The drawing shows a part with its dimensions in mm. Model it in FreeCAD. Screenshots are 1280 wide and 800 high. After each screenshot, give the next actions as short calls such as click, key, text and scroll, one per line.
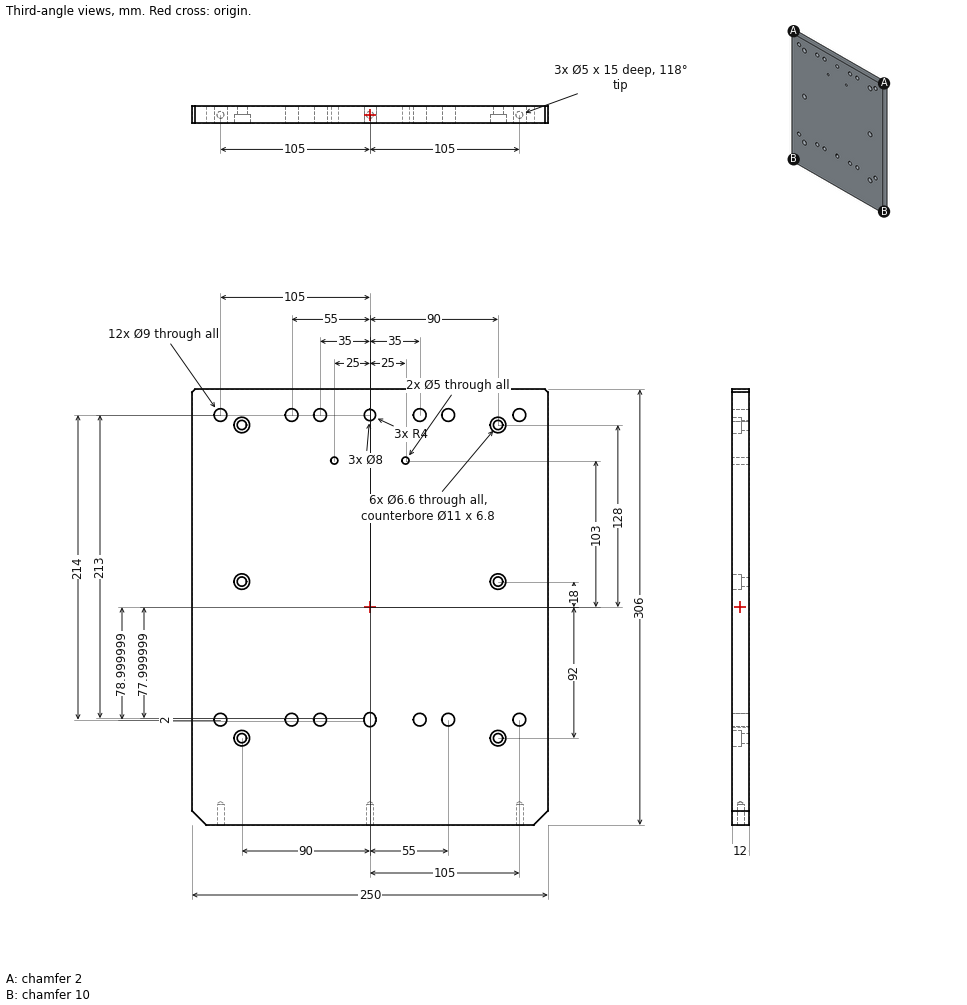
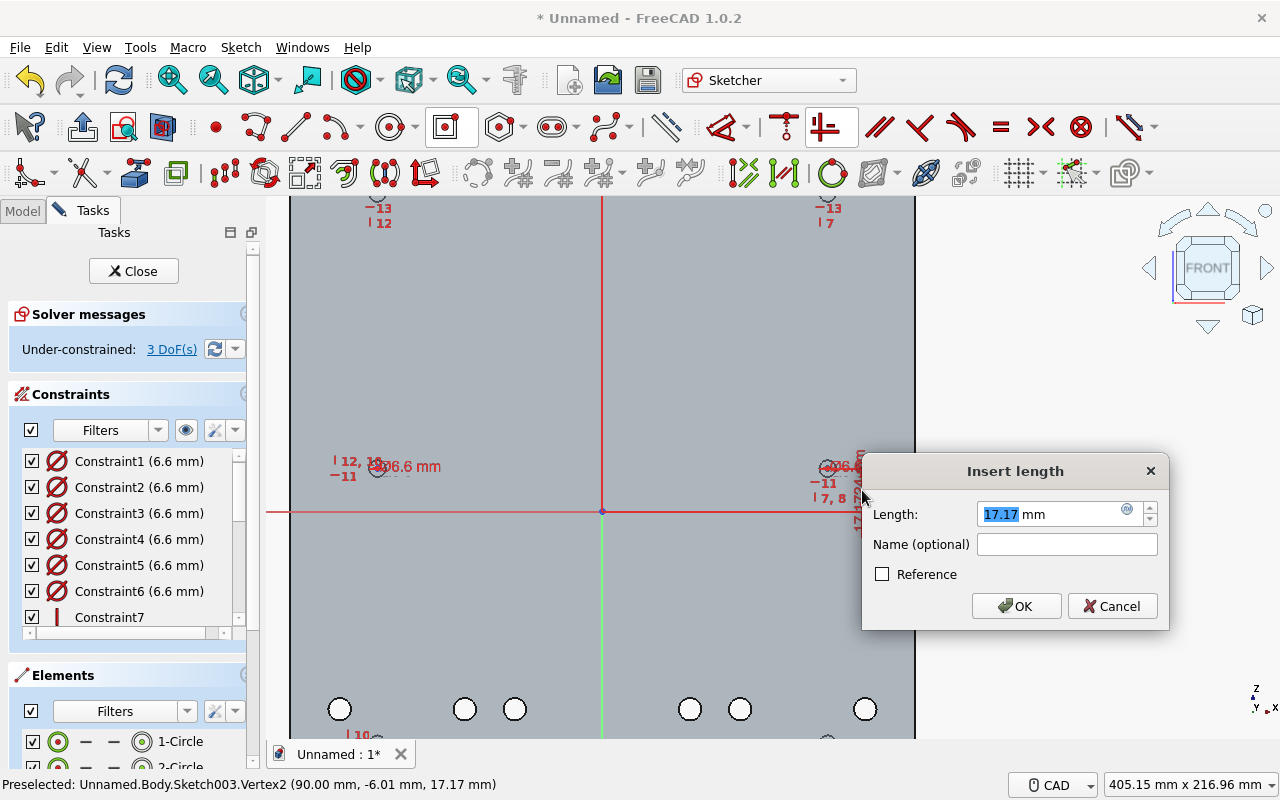
text(18)
key(Return)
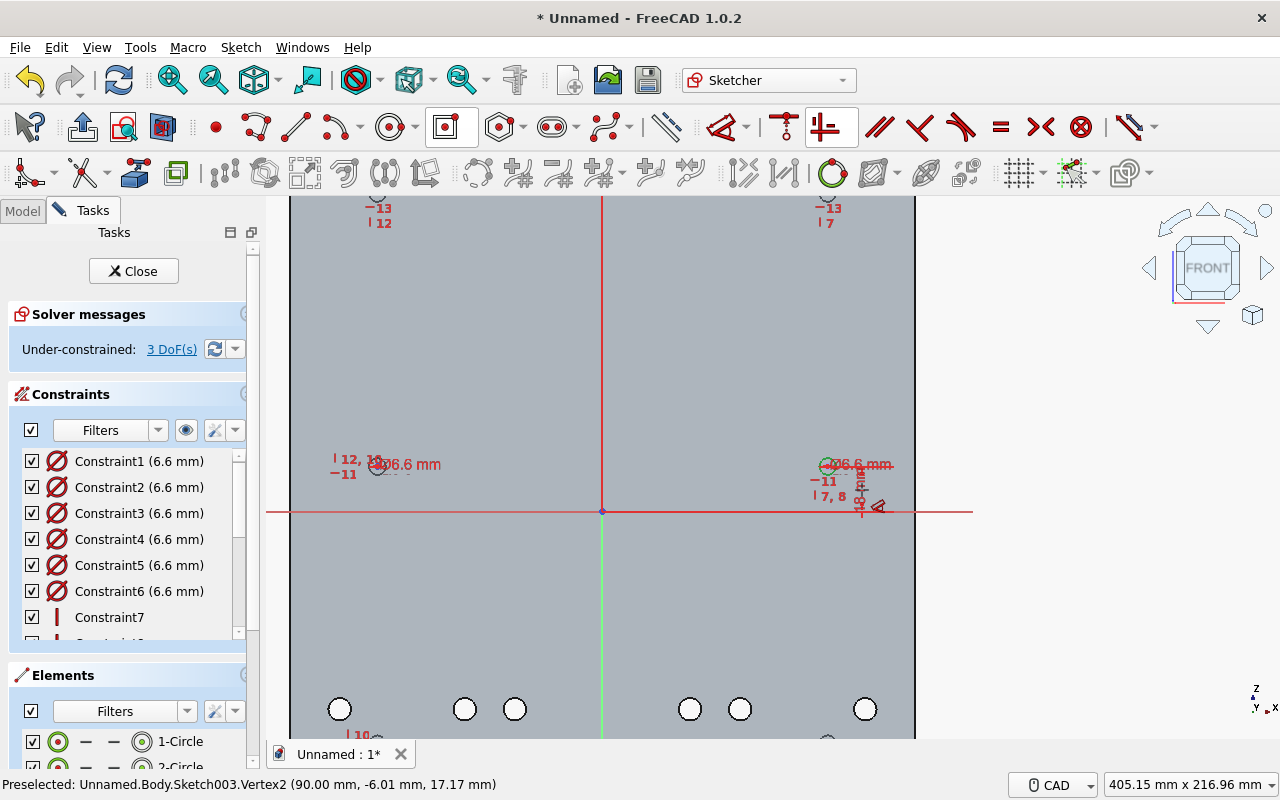
scroll(829, 469, down, 3)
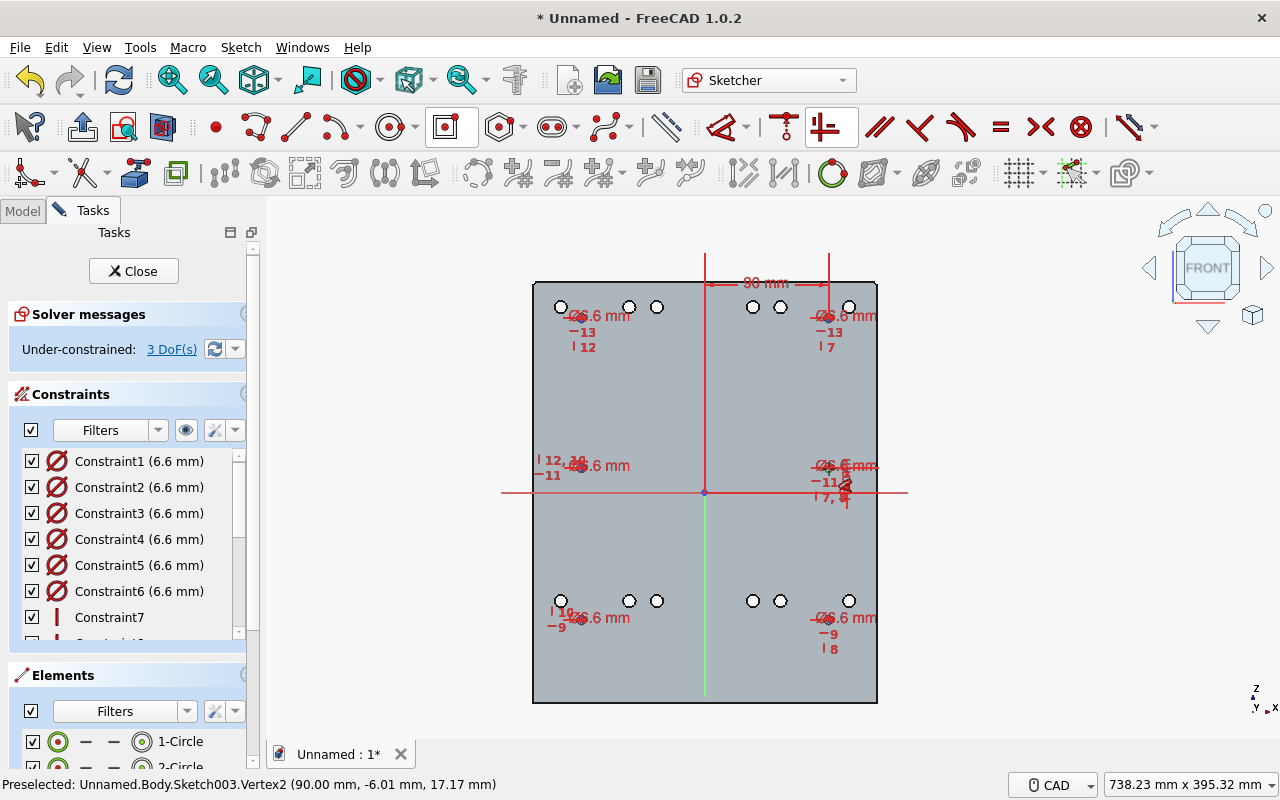
click(829, 620)
click(863, 556)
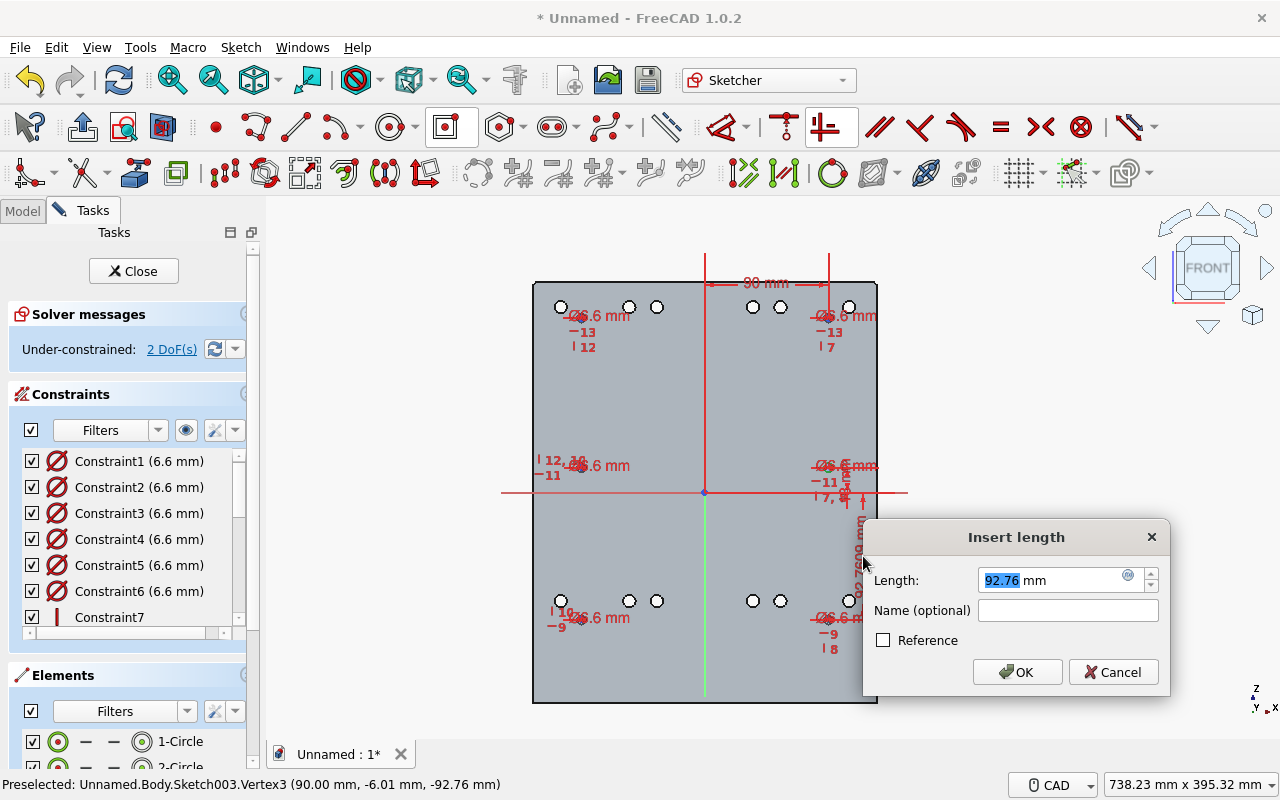
text(92)
key(Return)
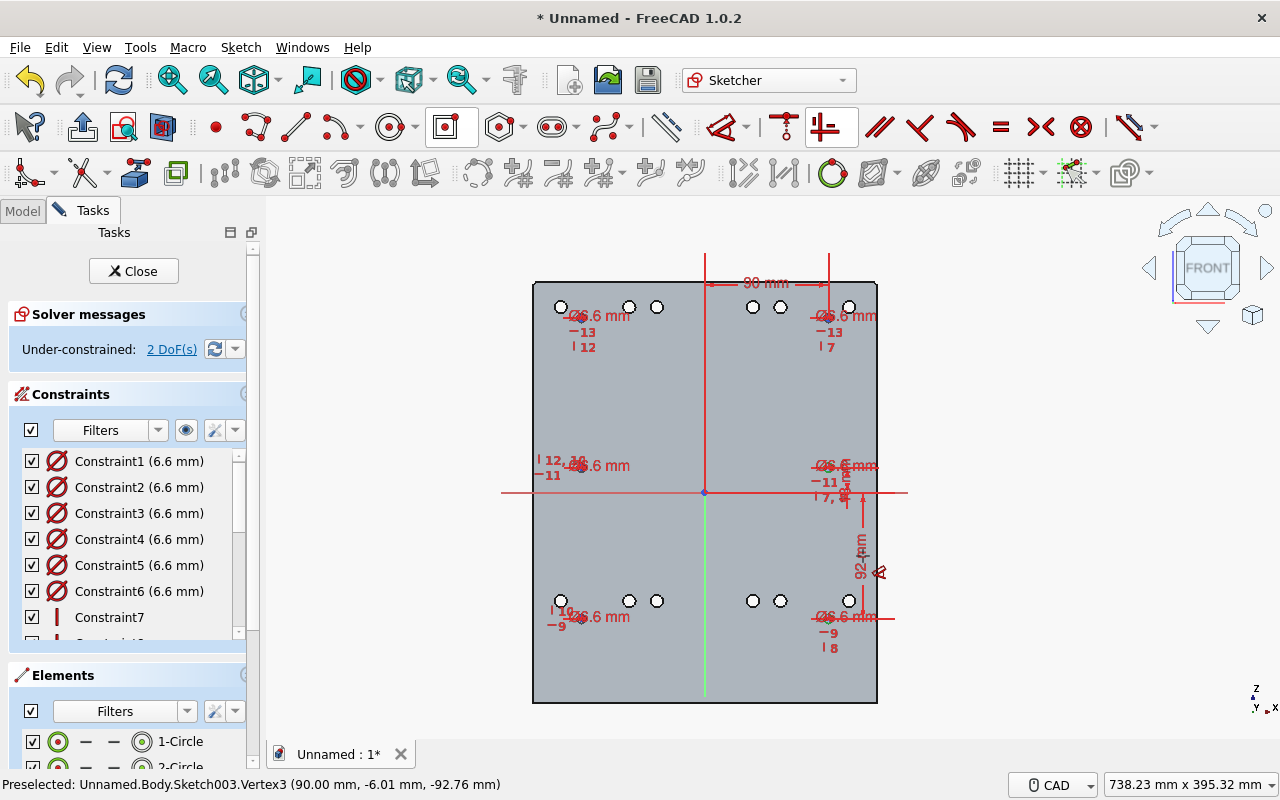
click(581, 619)
click(643, 653)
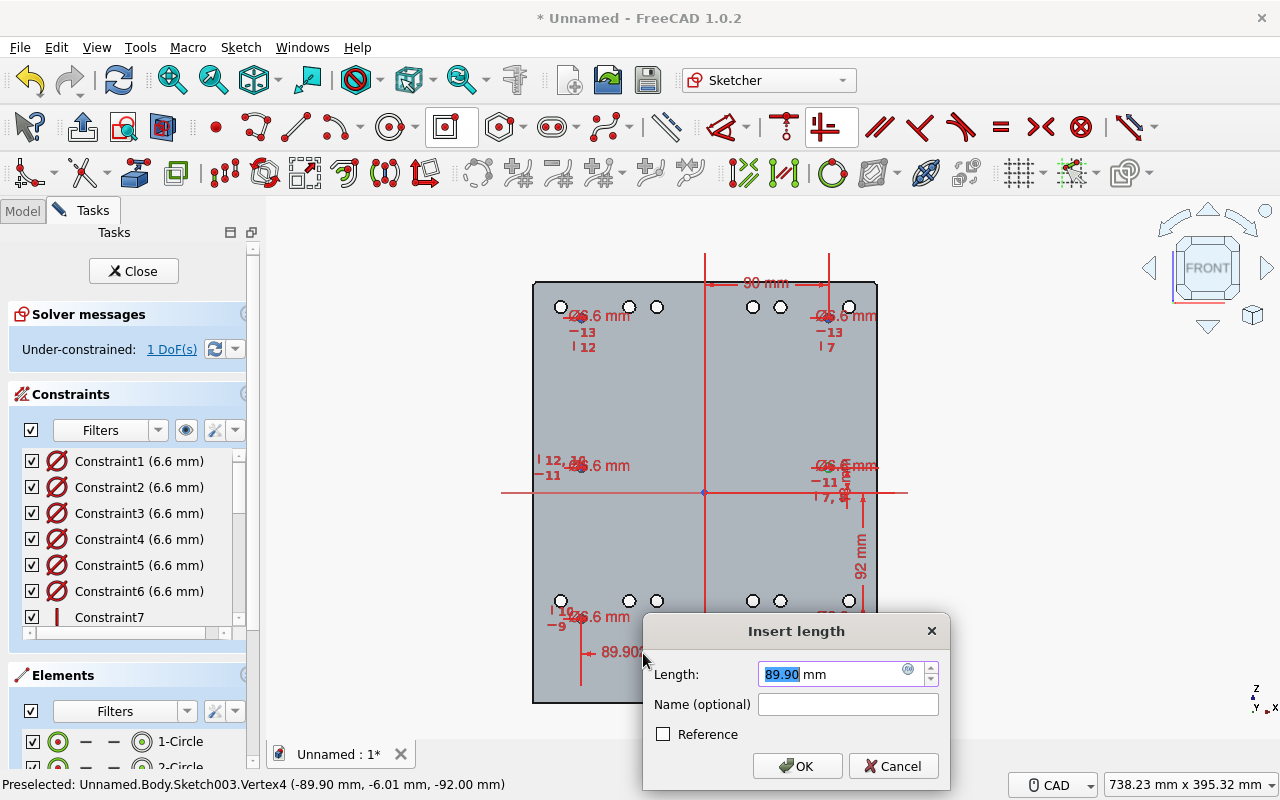
text(90)
key(Return)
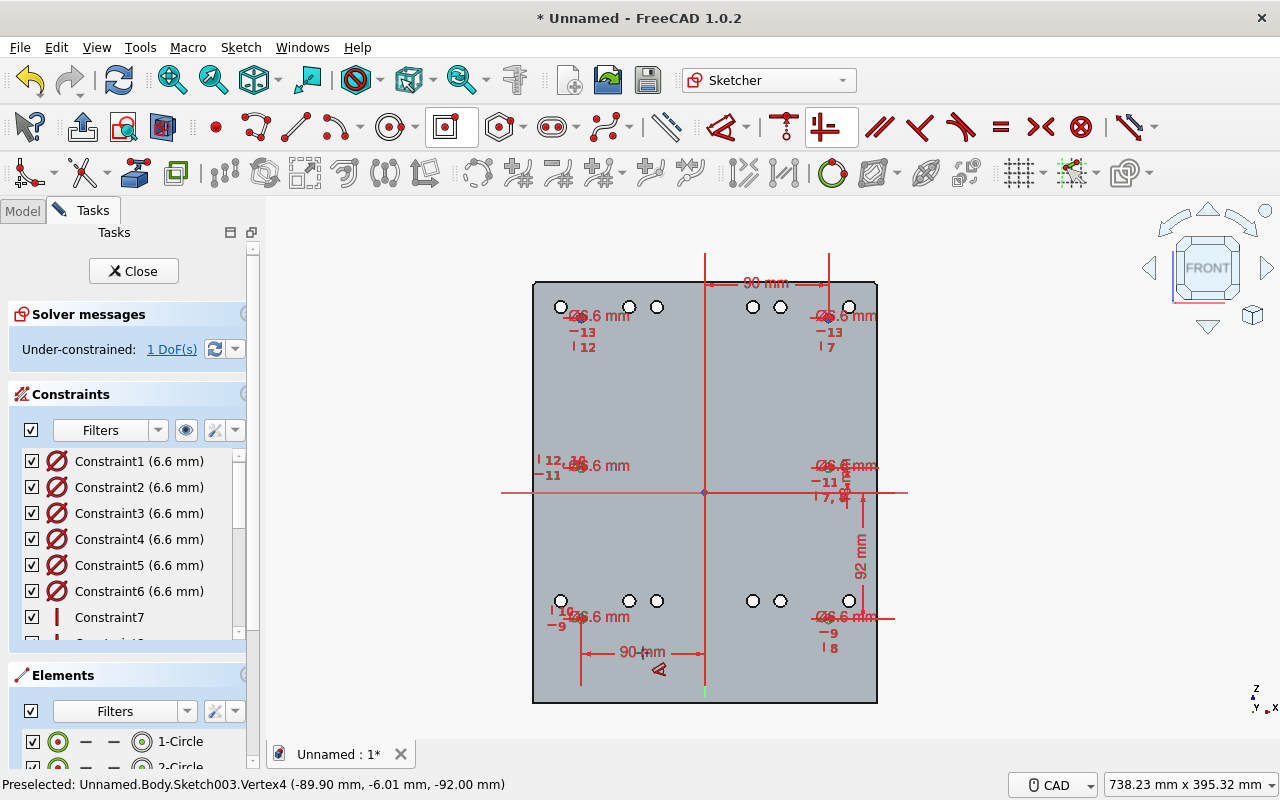
click(829, 318)
click(863, 405)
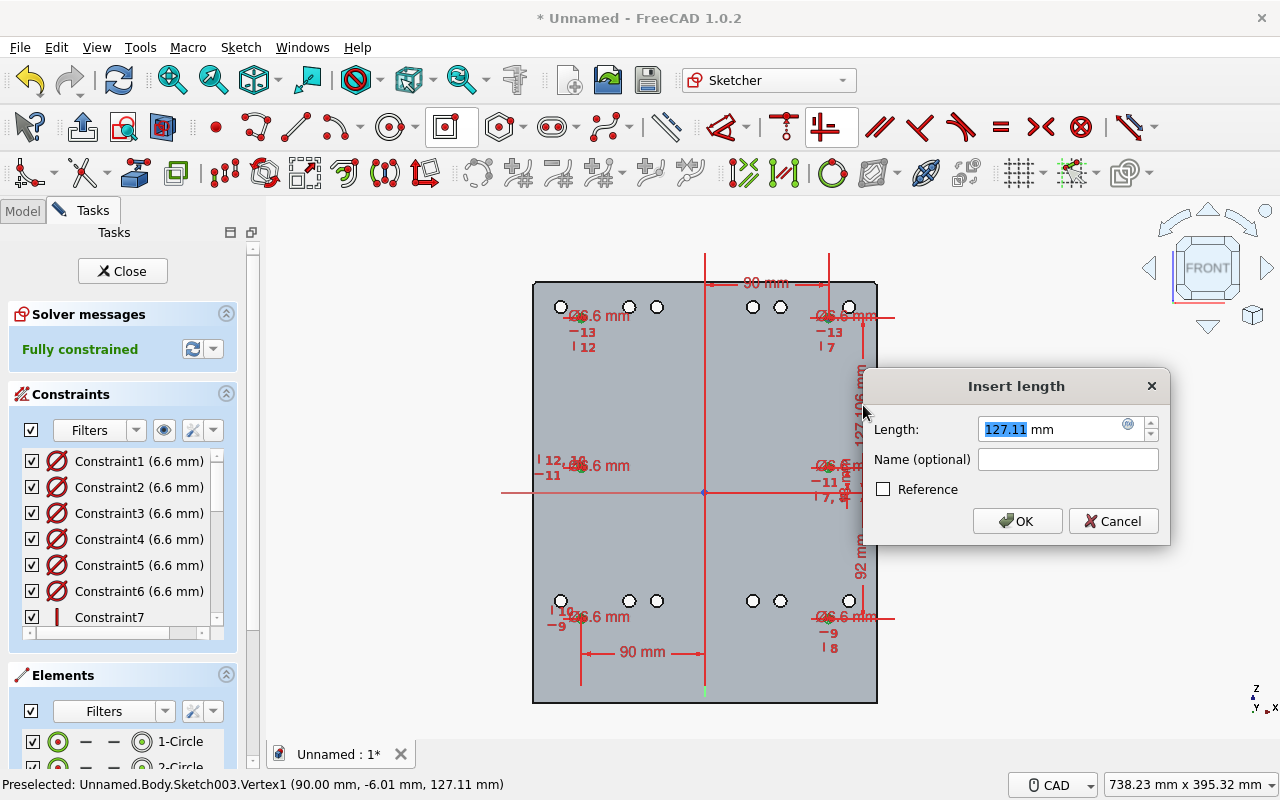
text(128)
key(Return)
key(Escape)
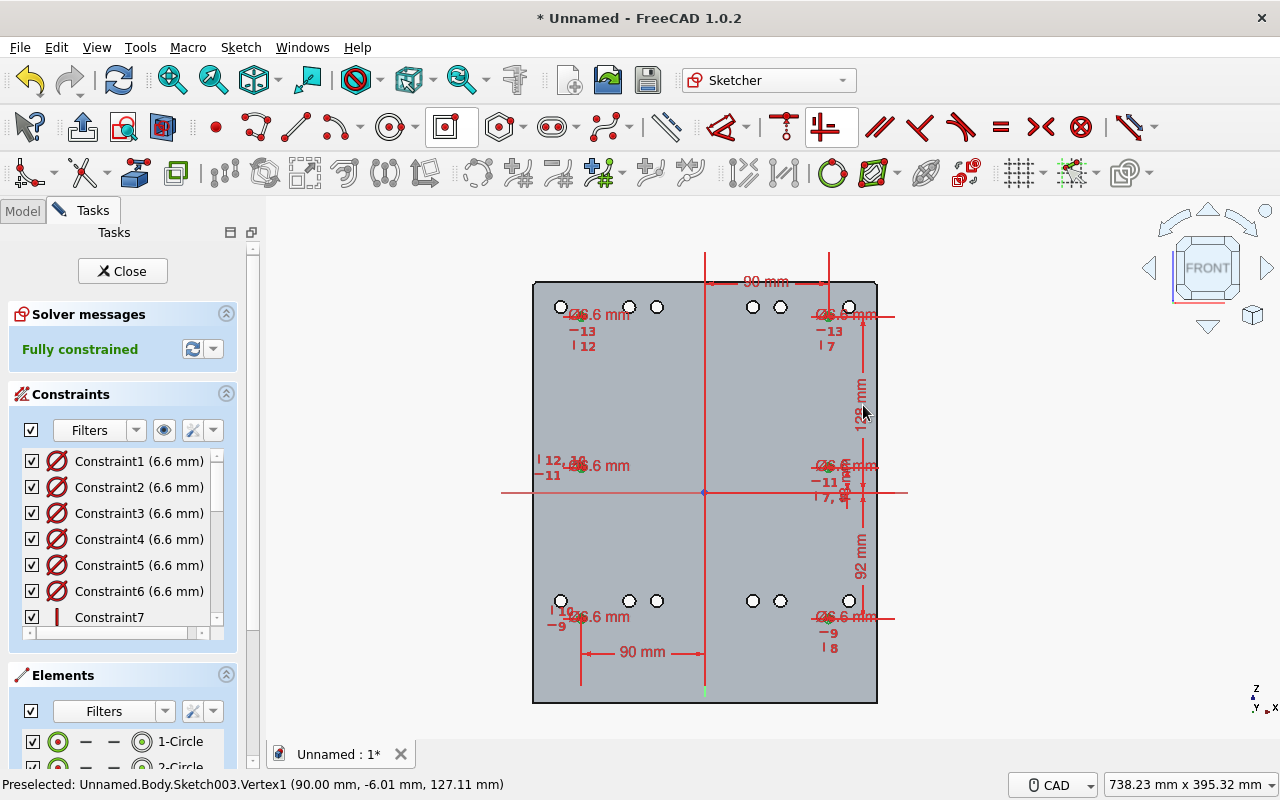
click(123, 271)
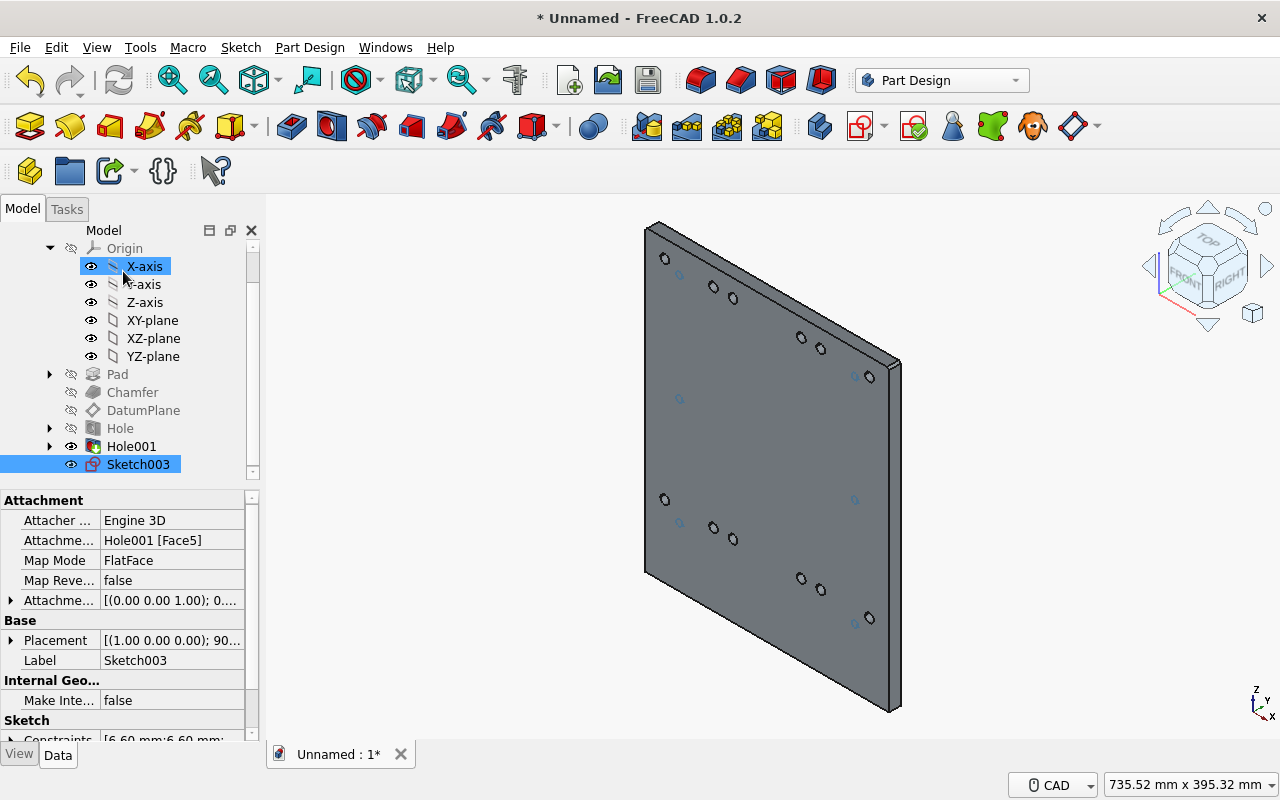
click(332, 126)